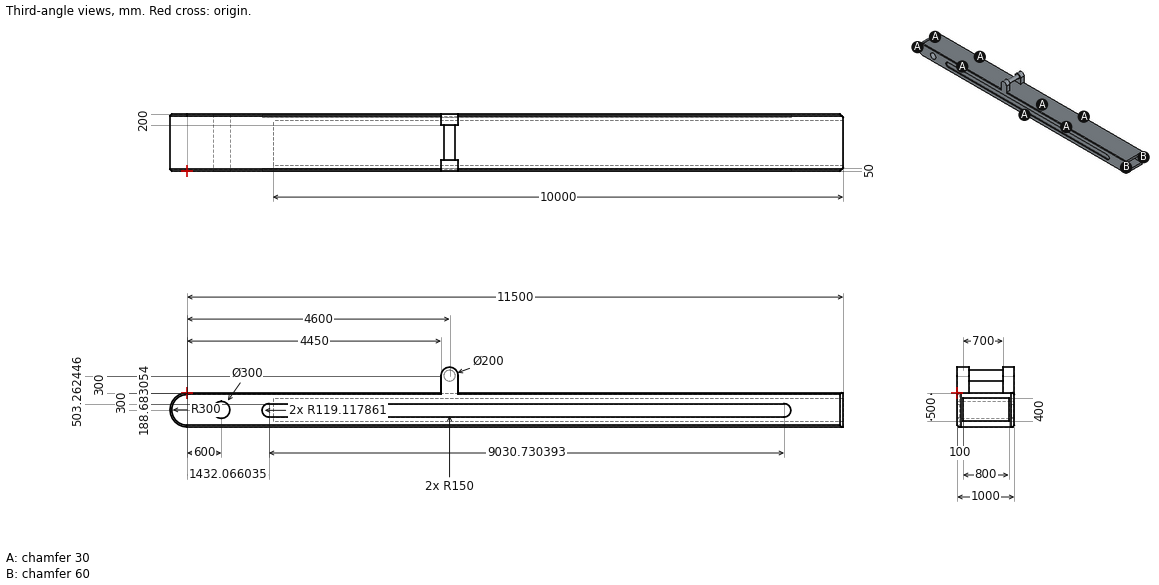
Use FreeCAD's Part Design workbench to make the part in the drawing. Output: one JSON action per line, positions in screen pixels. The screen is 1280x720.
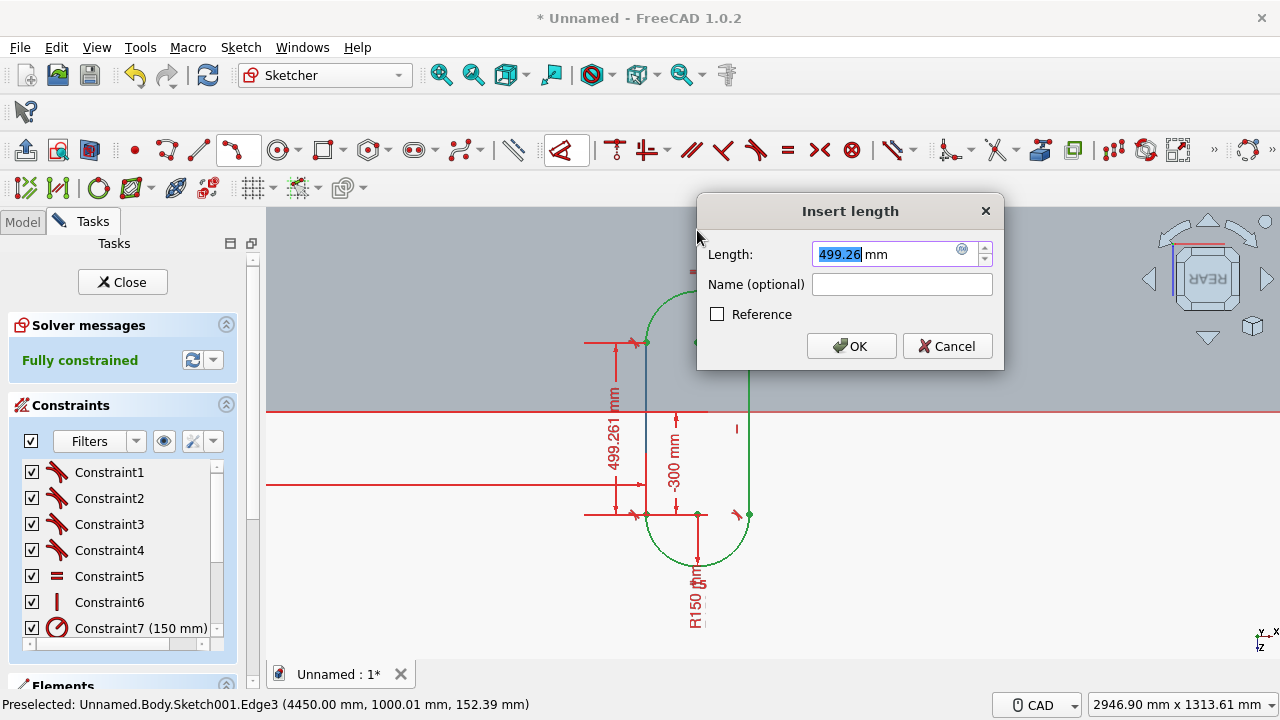
{"action": "type", "text": "503.262446"}
{"action": "key", "text": "Return"}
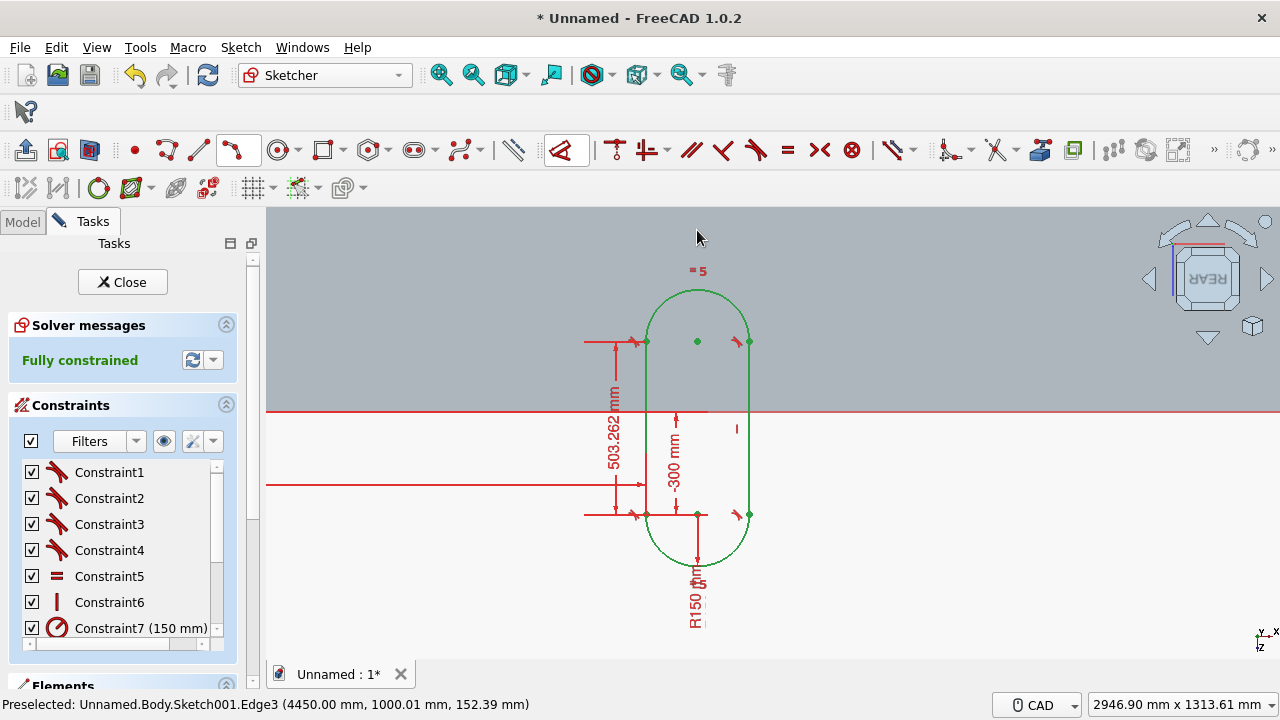
{"action": "left_click", "coordinate": [123, 282]}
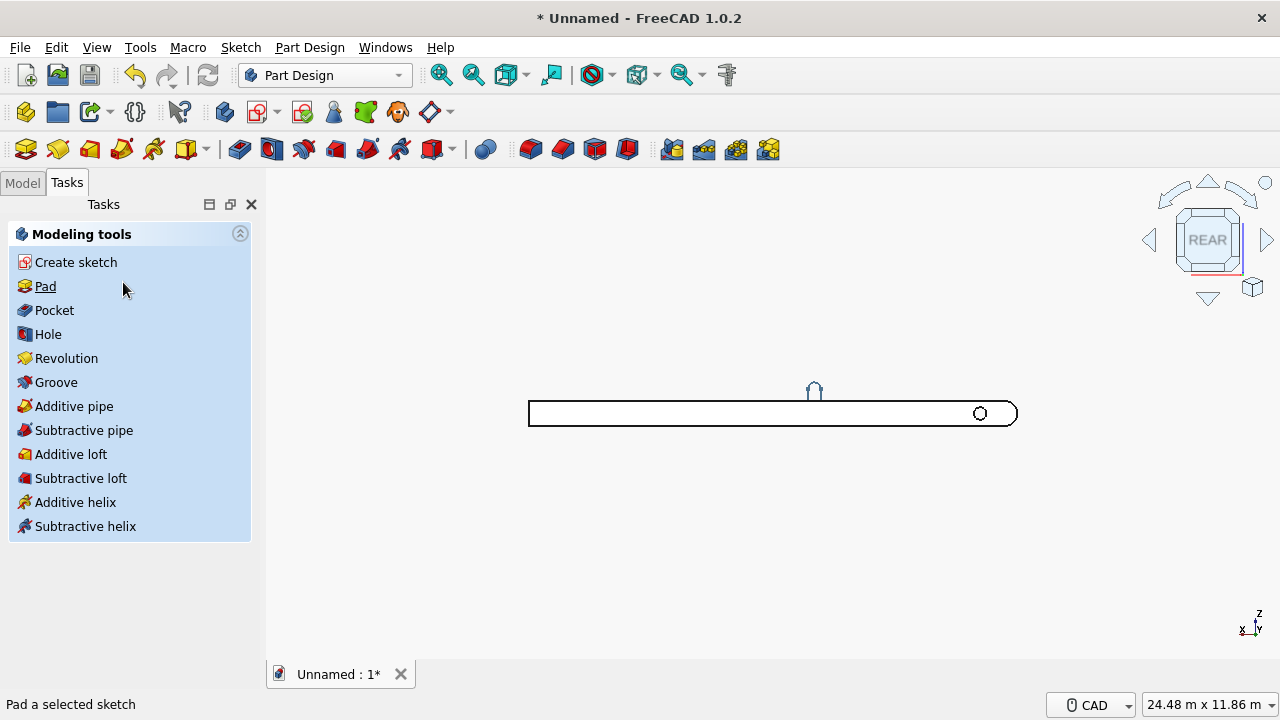
{"action": "left_click", "coordinate": [26, 150]}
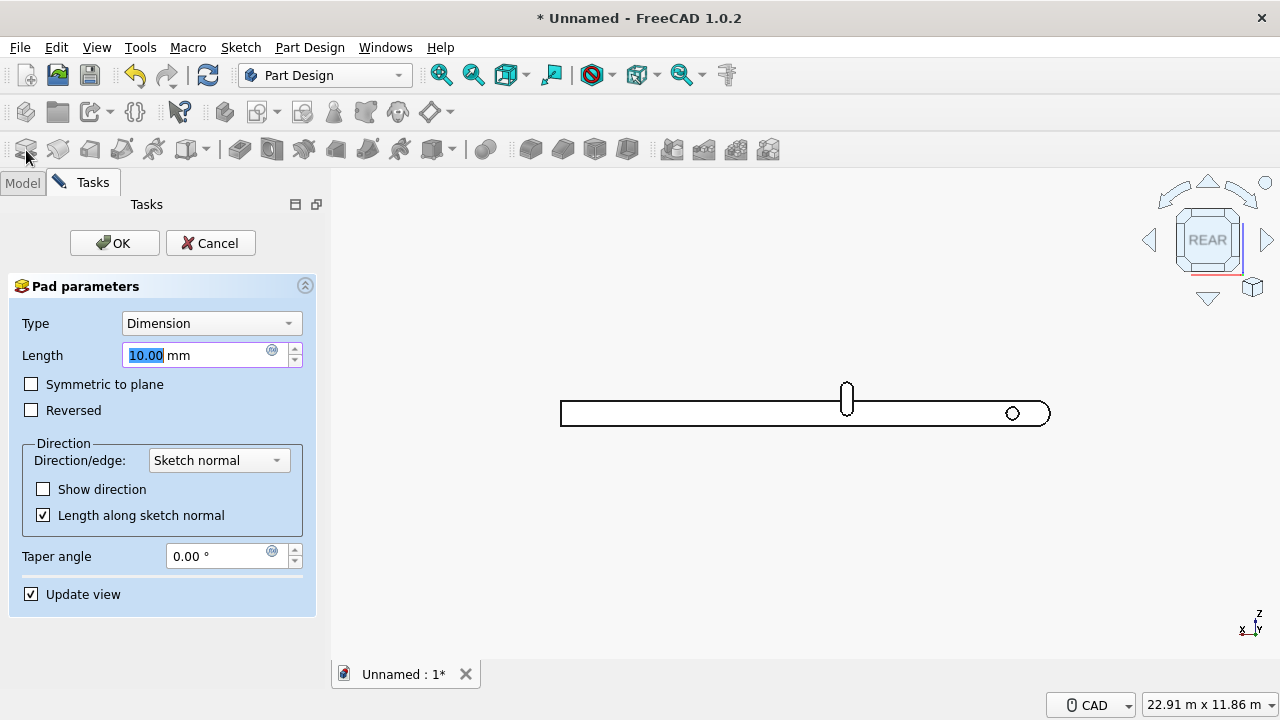
{"action": "type", "text": "200"}
{"action": "key", "text": "Tab"}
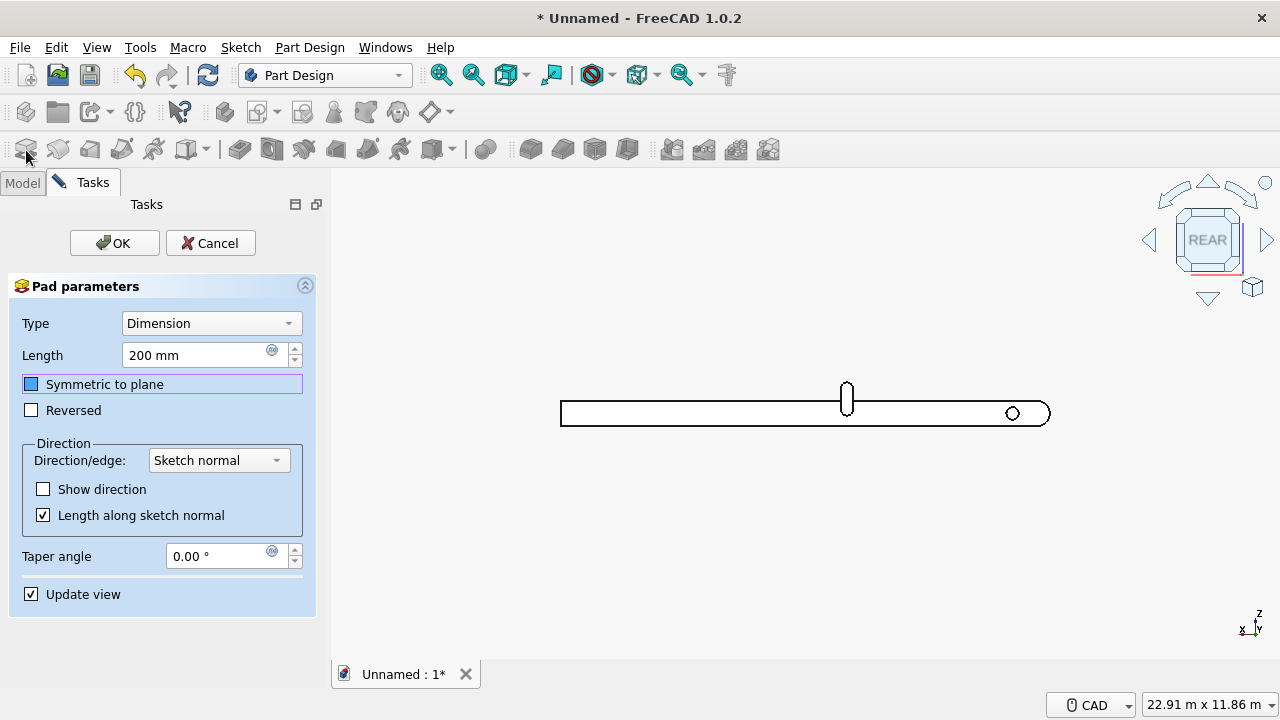
{"action": "left_click", "coordinate": [30, 410]}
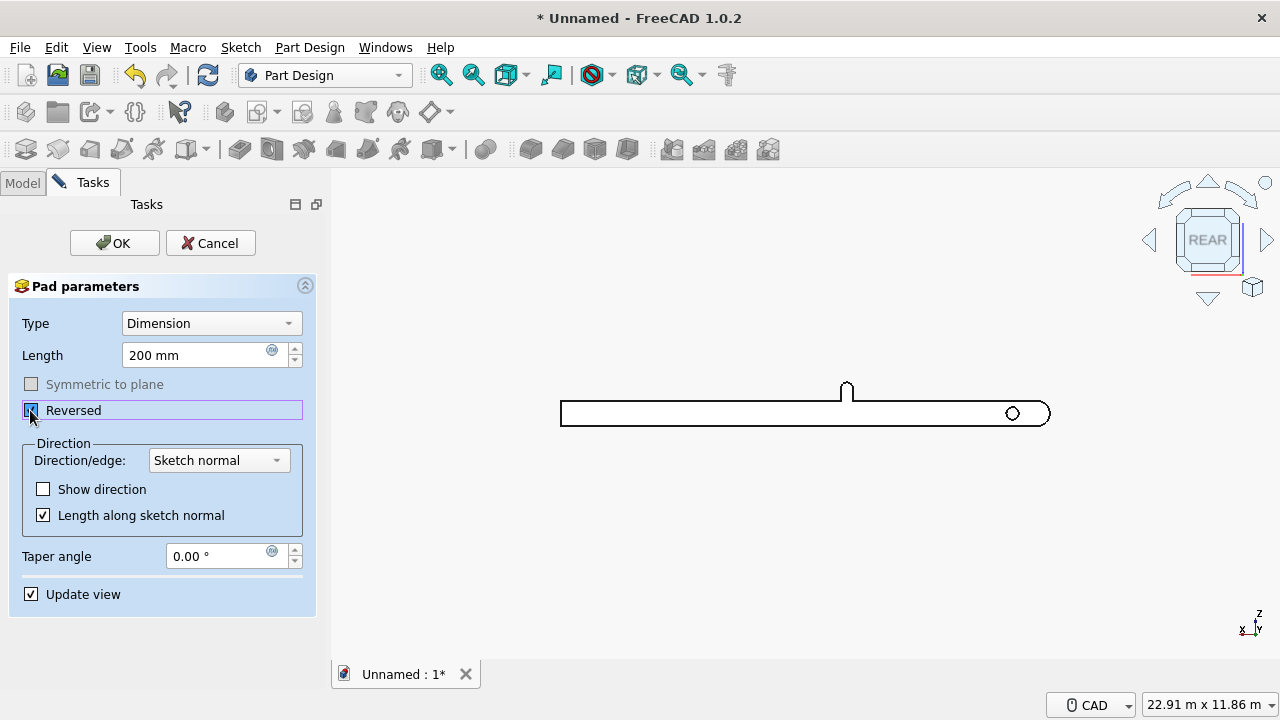
{"action": "left_click", "coordinate": [115, 243]}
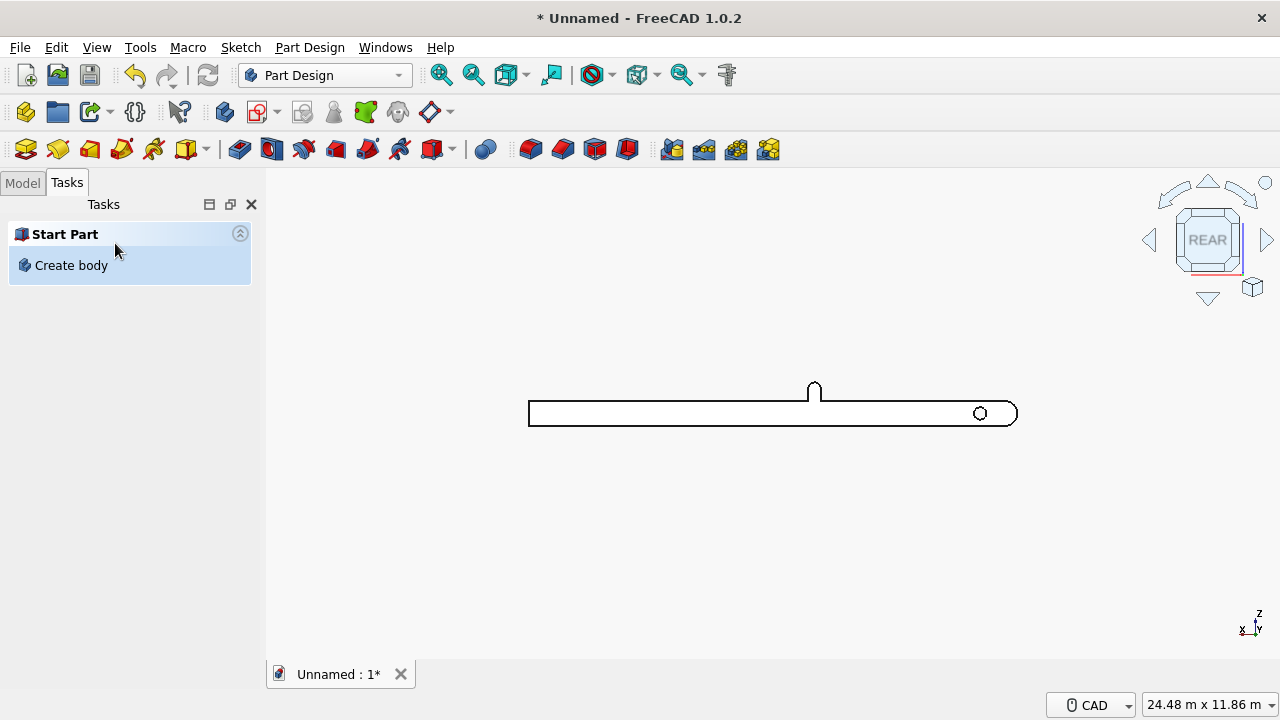
{"action": "left_click", "coordinate": [23, 182]}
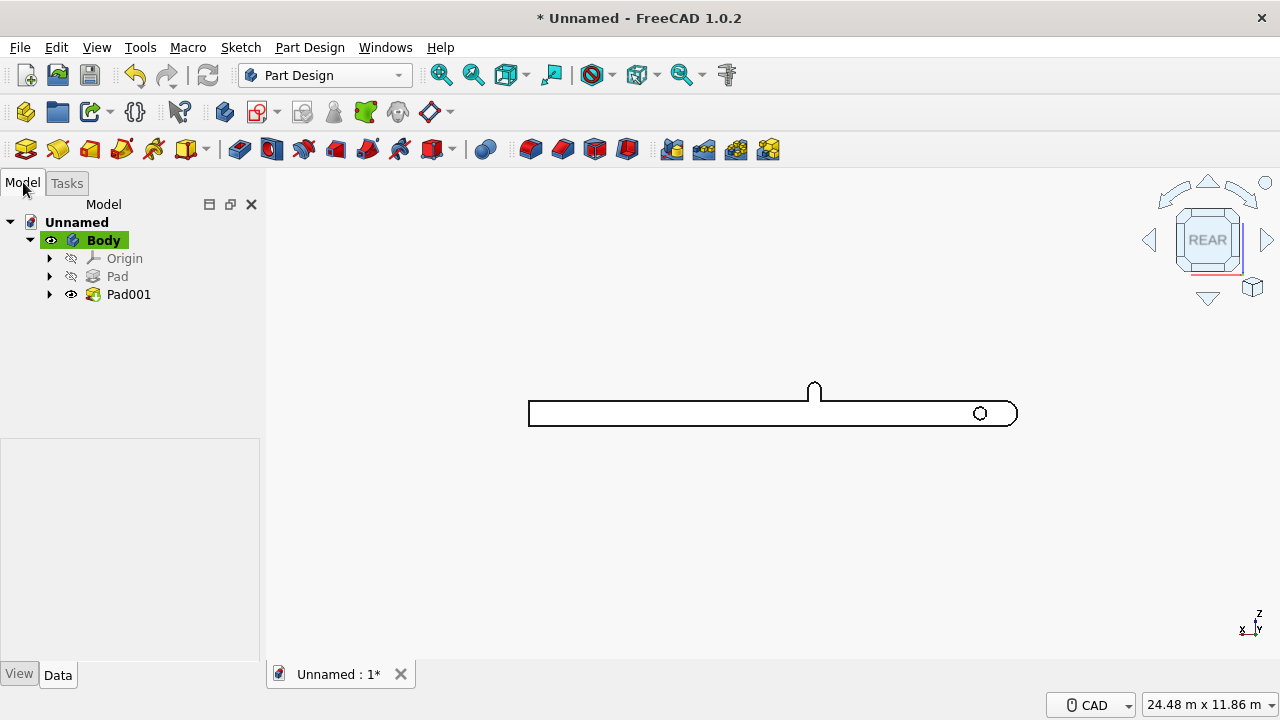
{"action": "left_click", "coordinate": [50, 258]}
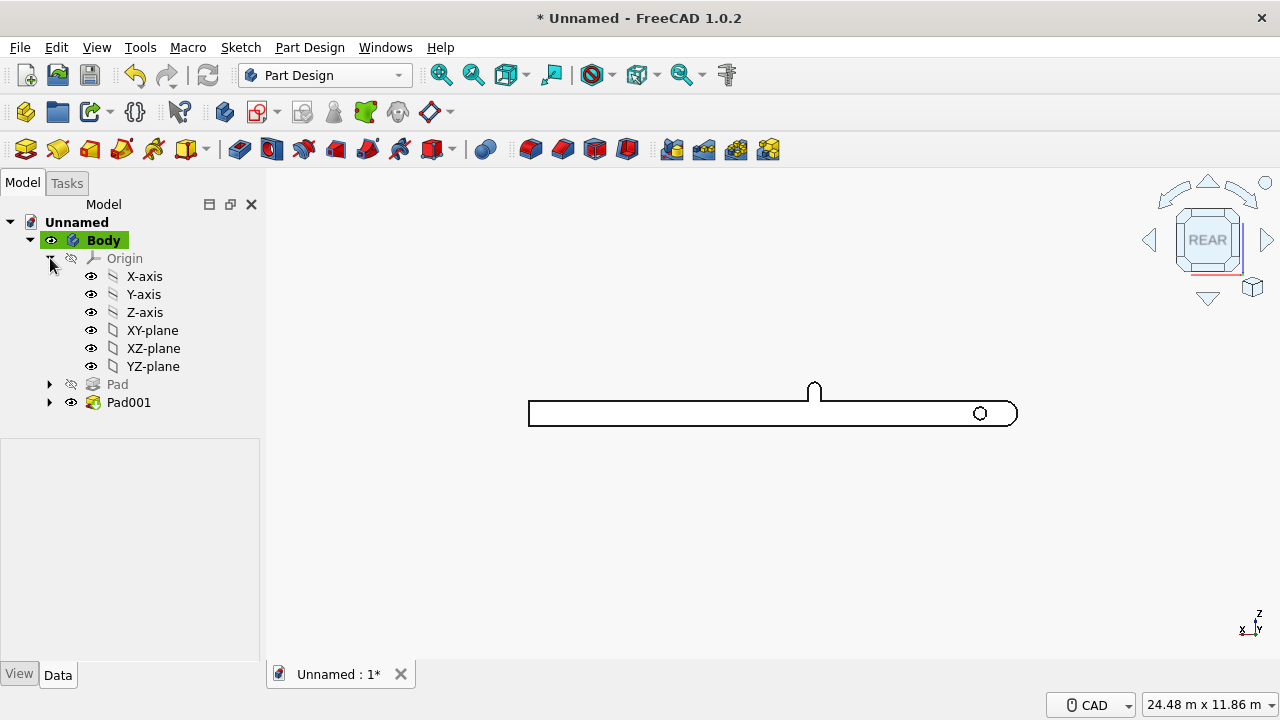
{"action": "left_click", "coordinate": [136, 348]}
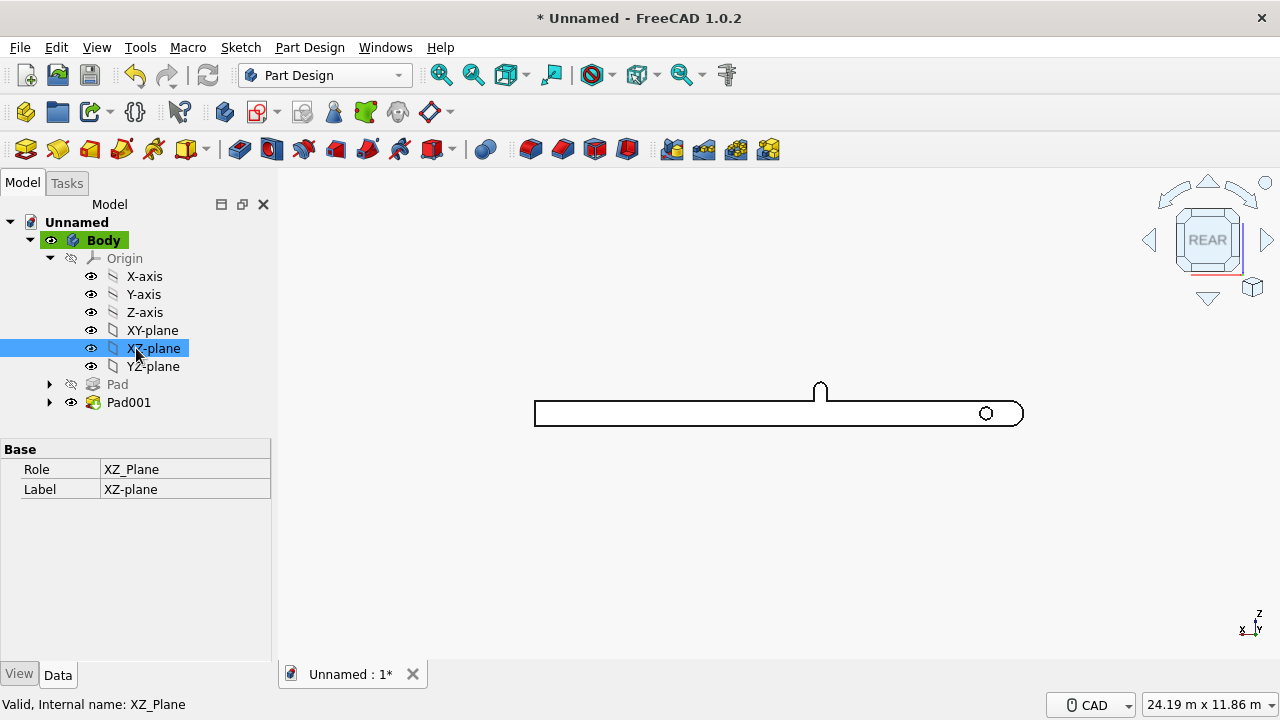
{"action": "left_click", "coordinate": [430, 112]}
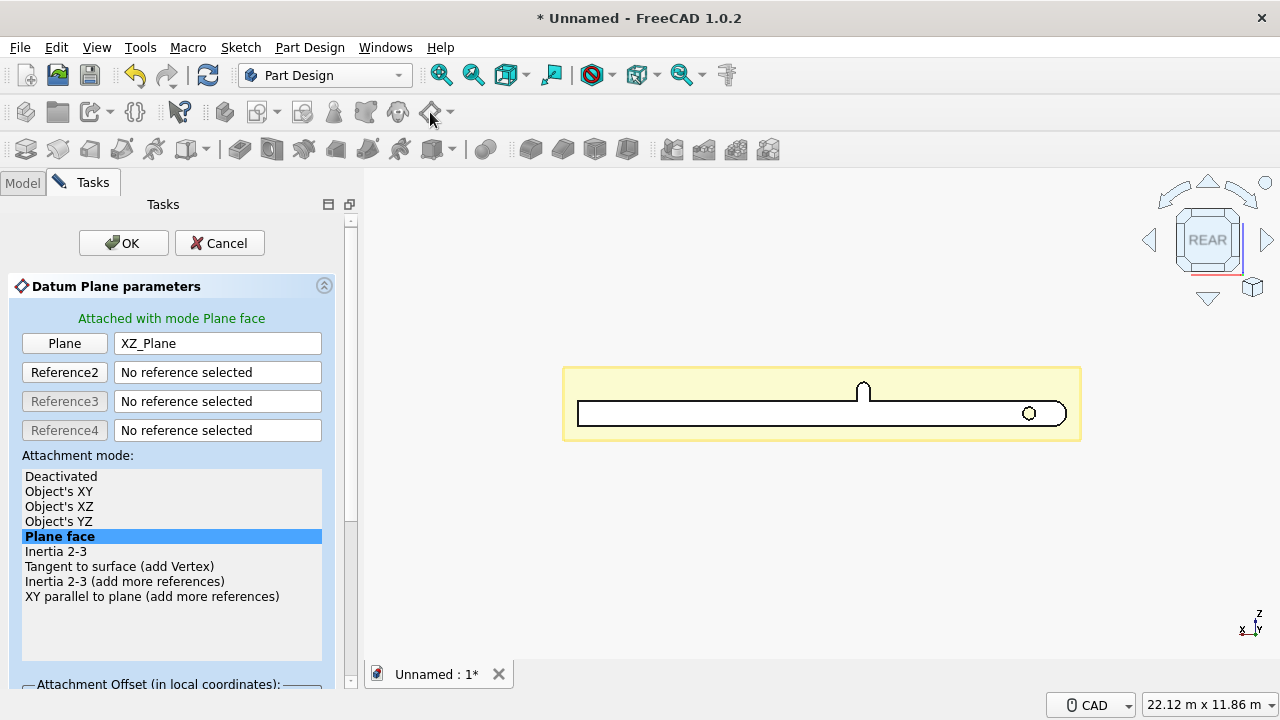
{"action": "scroll", "coordinate": [351, 451], "scroll_direction": "down", "scroll_amount": 3}